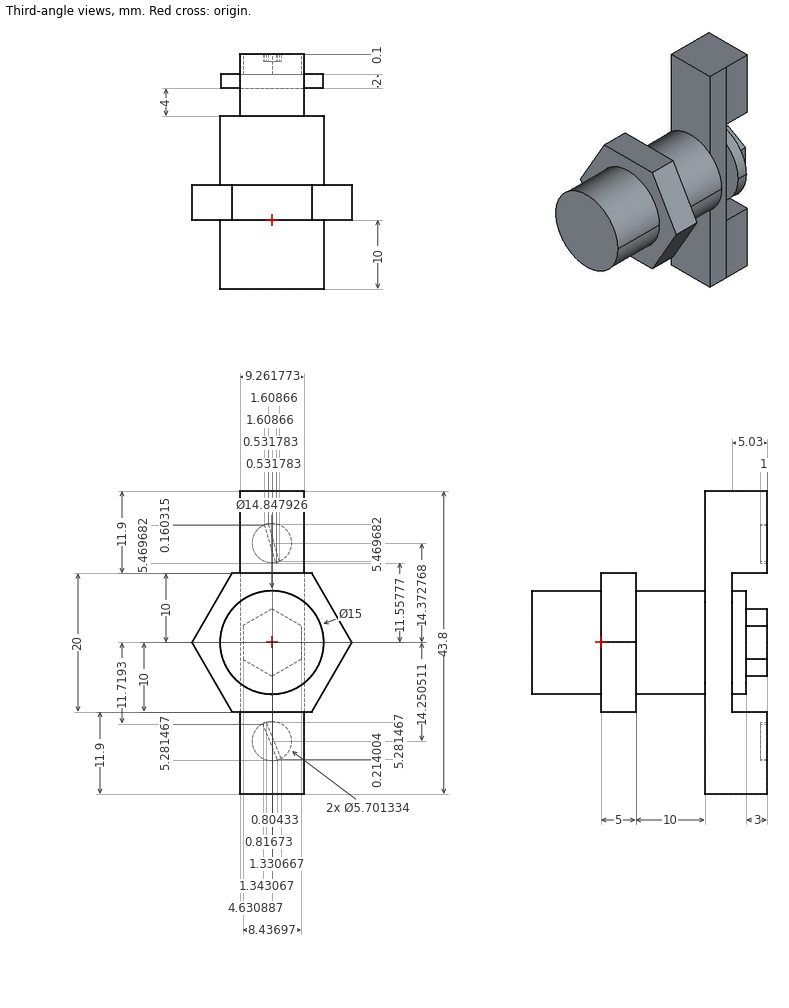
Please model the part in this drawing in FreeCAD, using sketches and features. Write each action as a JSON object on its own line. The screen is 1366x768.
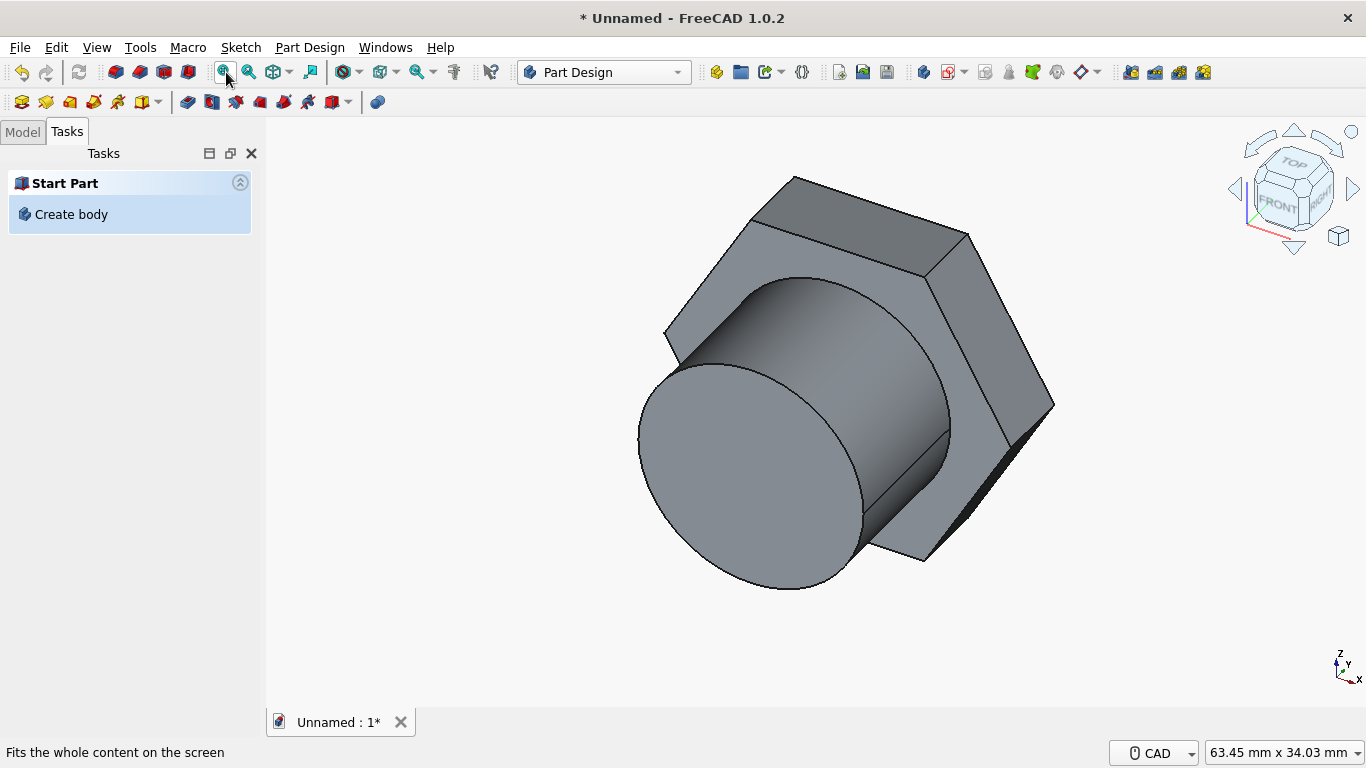
{"action": "left_click", "coordinate": [23, 131]}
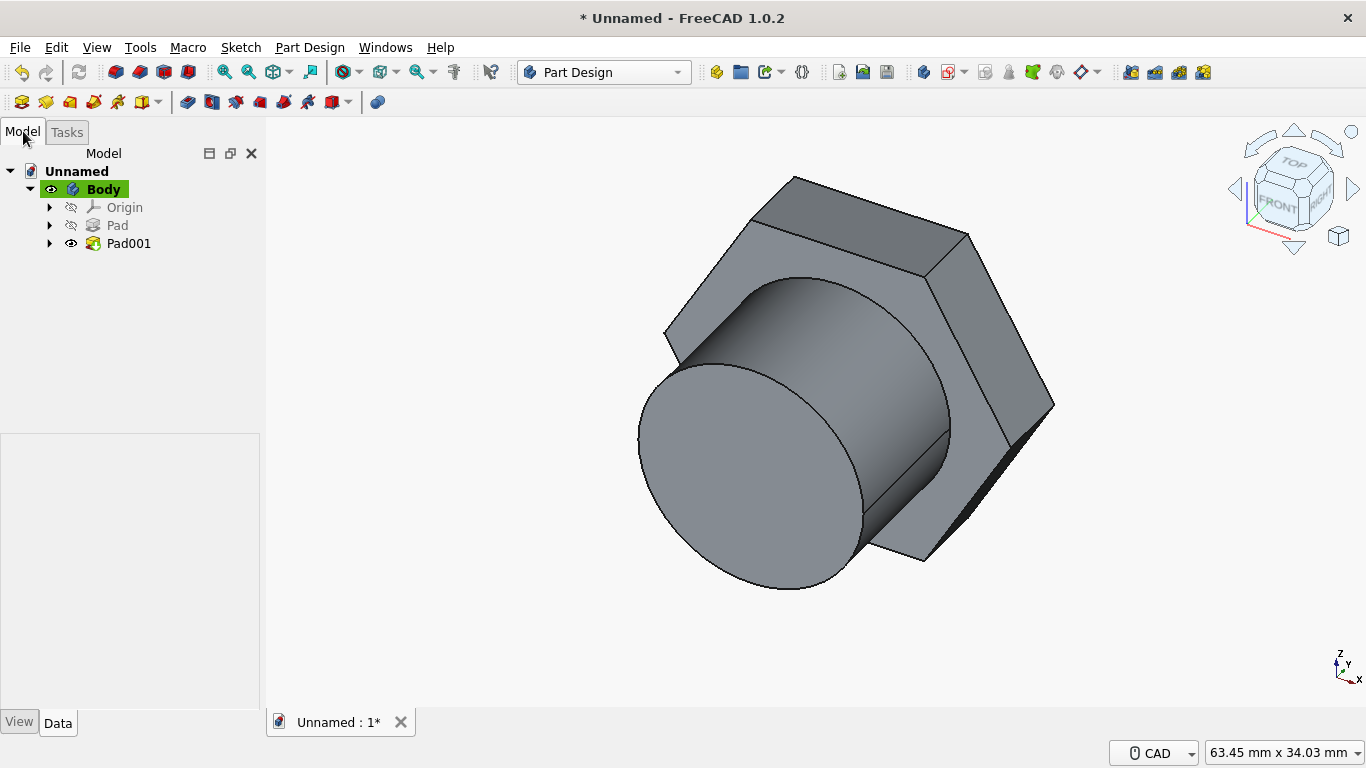
{"action": "left_click", "coordinate": [50, 207]}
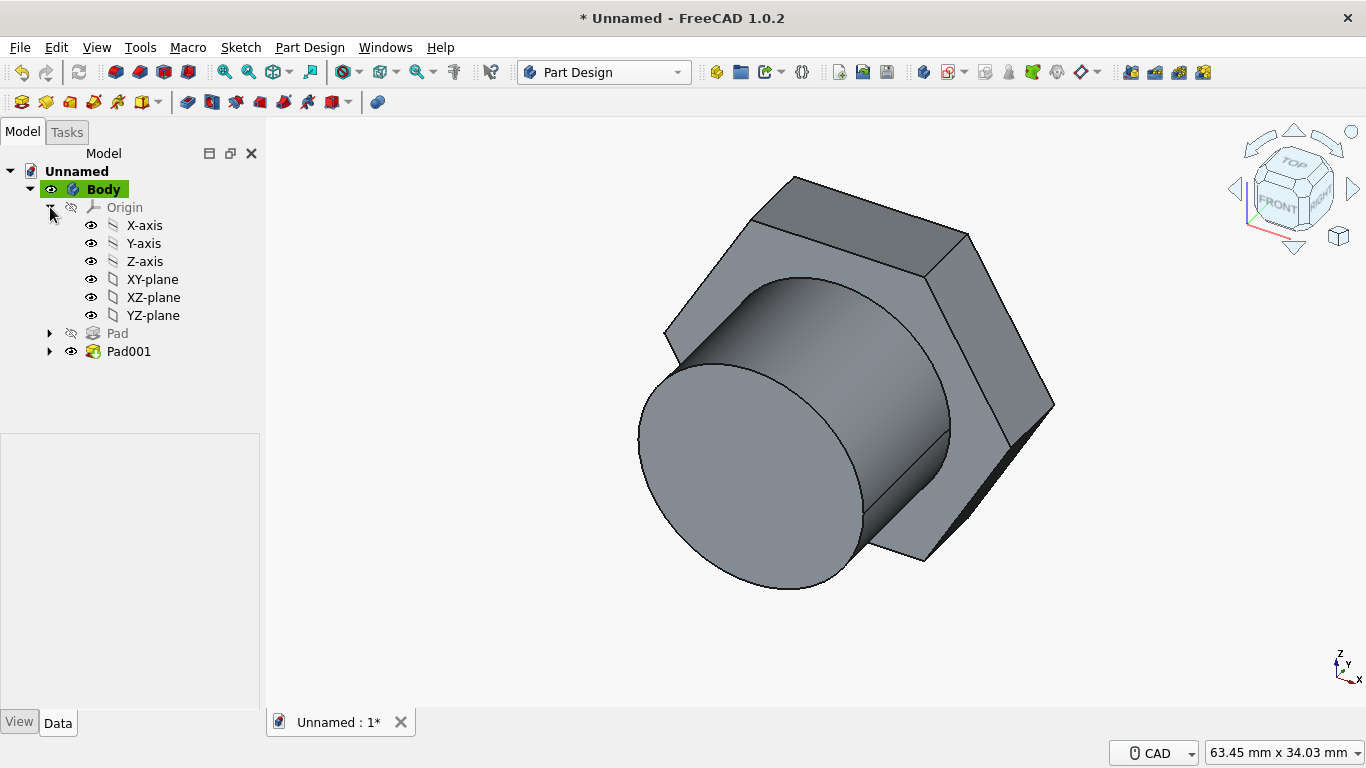
{"action": "left_click", "coordinate": [136, 297]}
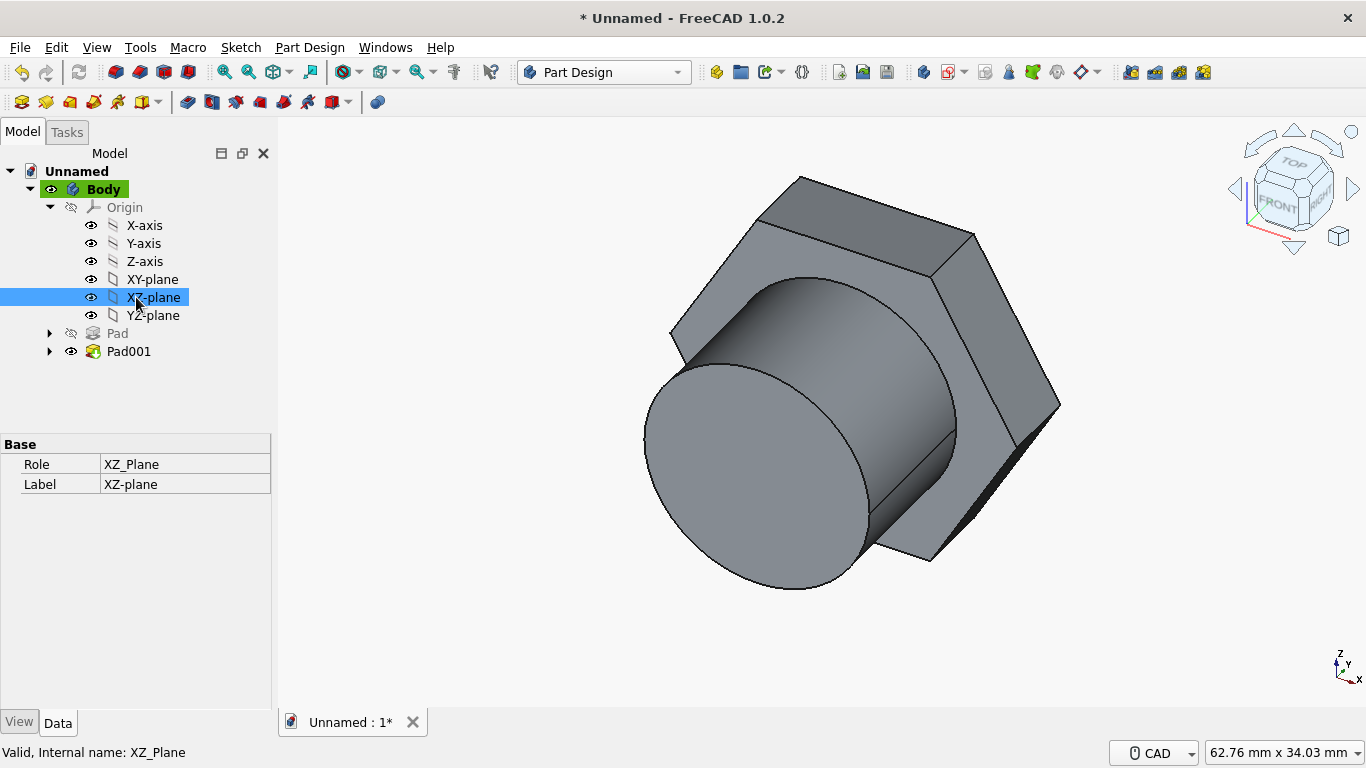
{"action": "left_click", "coordinate": [1082, 72]}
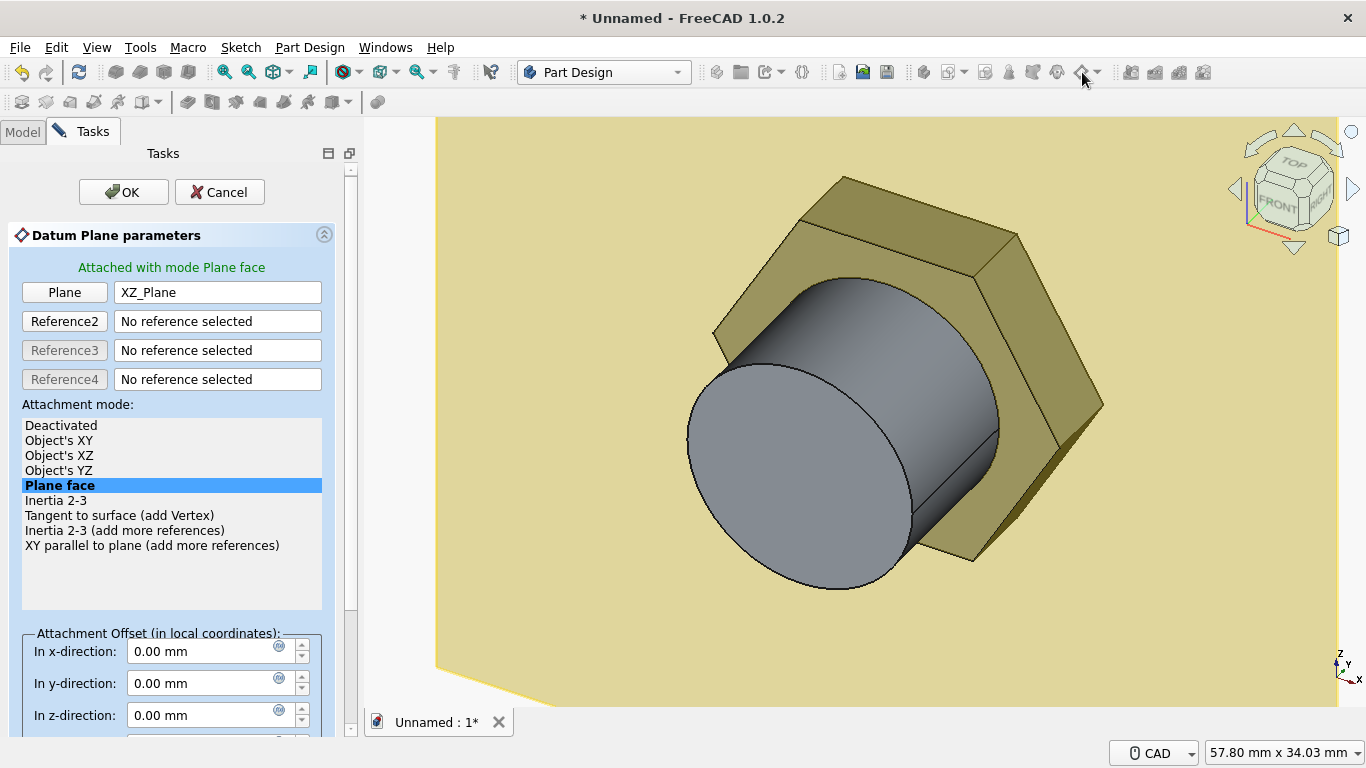
{"action": "triple_click", "coordinate": [210, 715]}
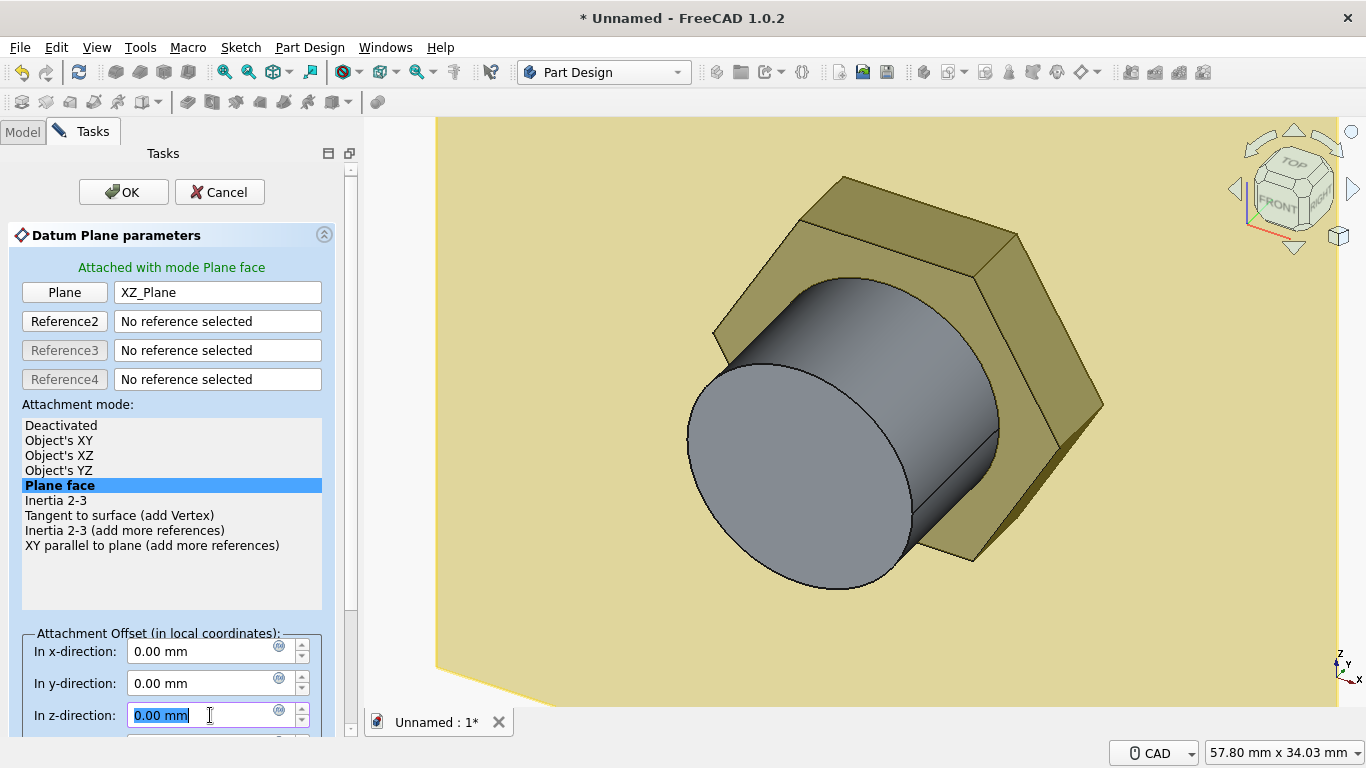
{"action": "type", "text": "-15"}
{"action": "key", "text": "Tab"}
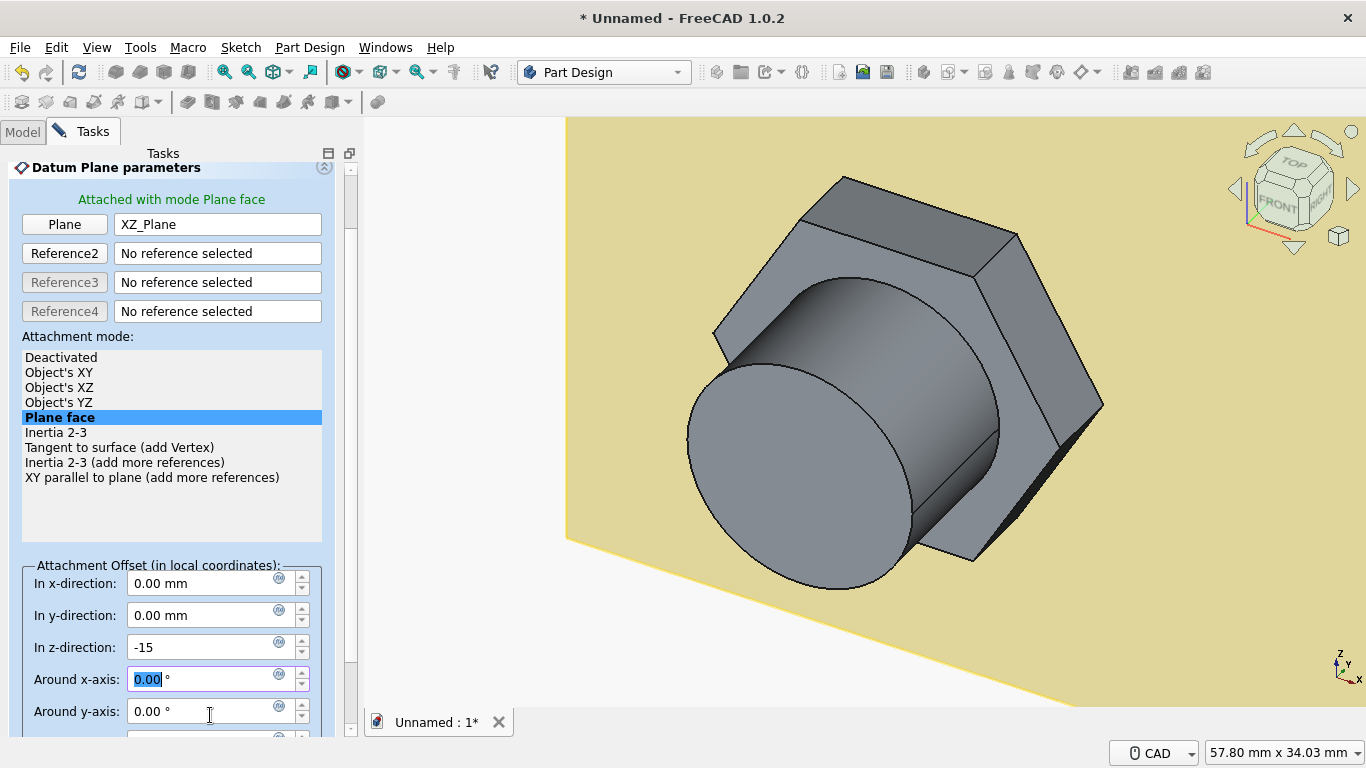
{"action": "scroll", "coordinate": [351, 450], "scroll_direction": "up", "scroll_amount": 2}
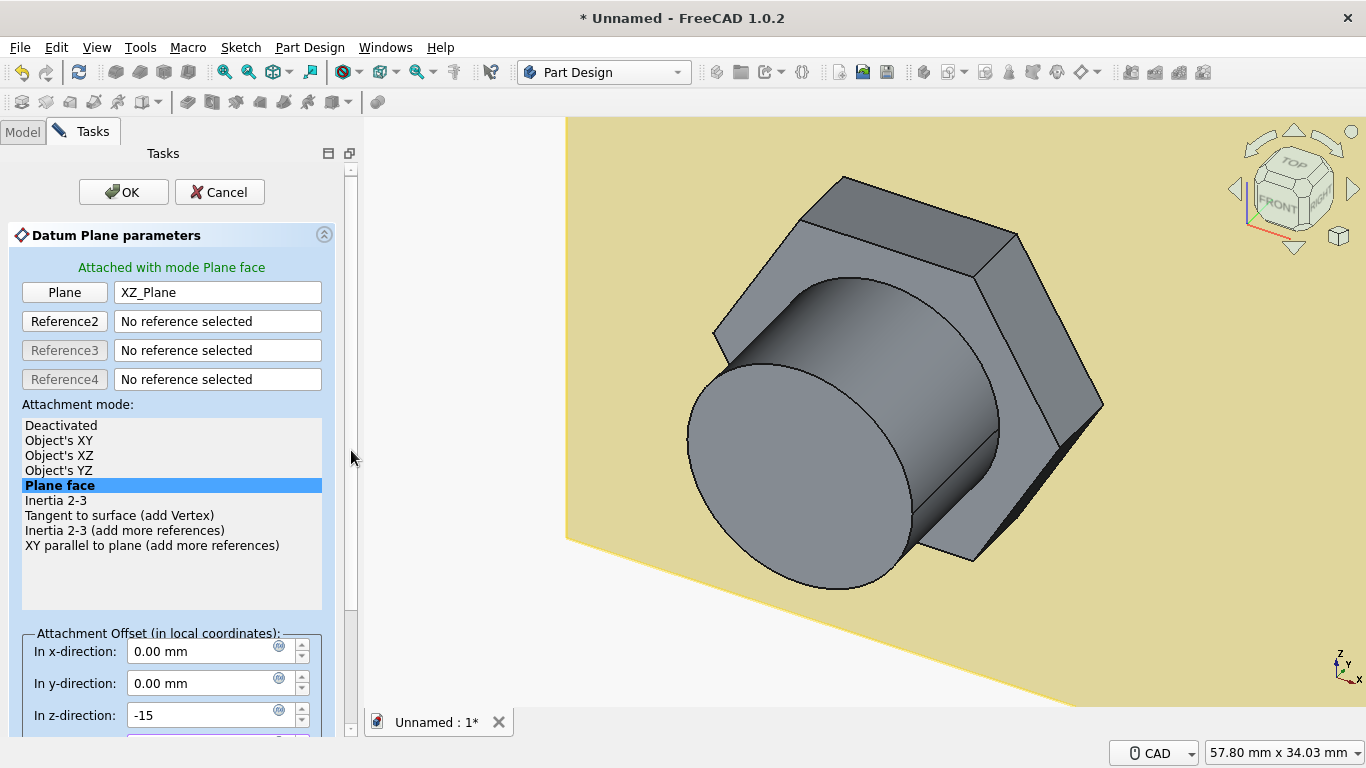
{"action": "left_click", "coordinate": [124, 192]}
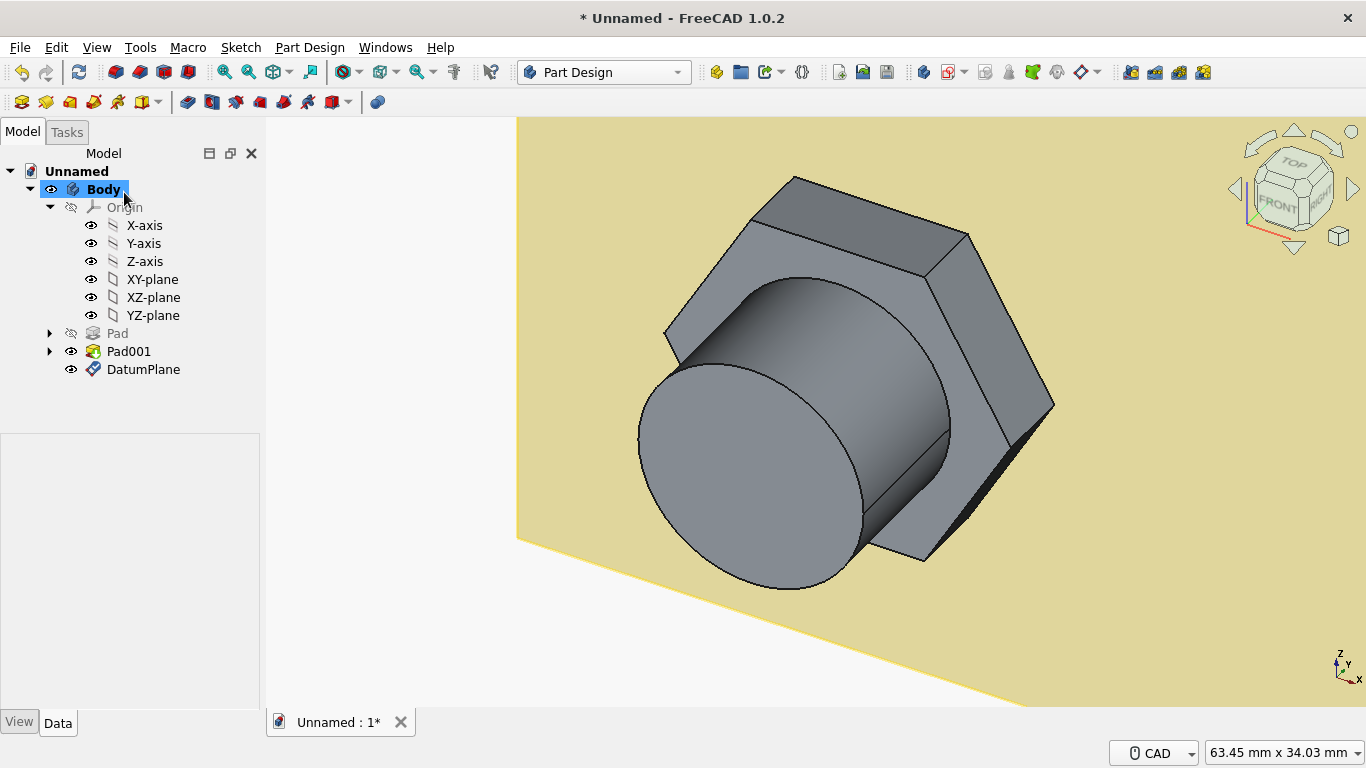
{"action": "left_click", "coordinate": [116, 369]}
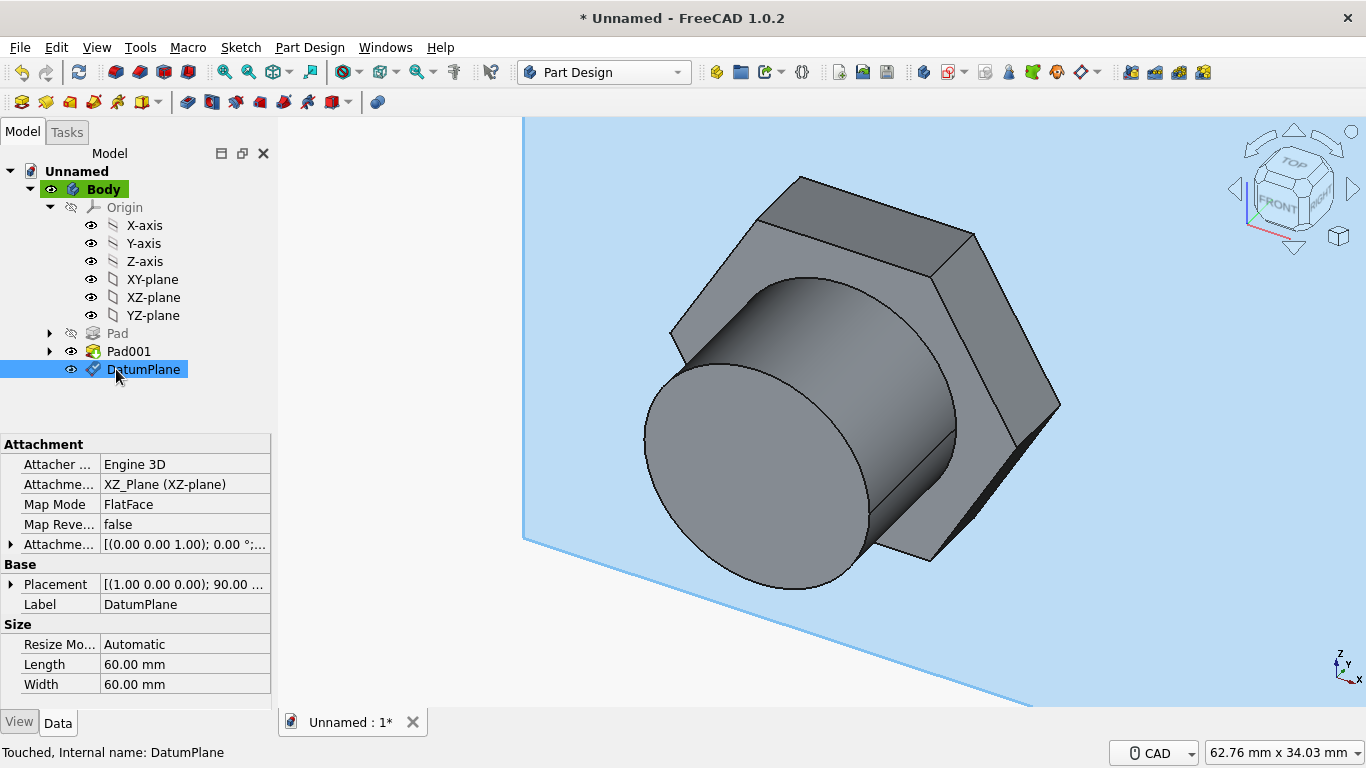
{"action": "left_click", "coordinate": [948, 72]}